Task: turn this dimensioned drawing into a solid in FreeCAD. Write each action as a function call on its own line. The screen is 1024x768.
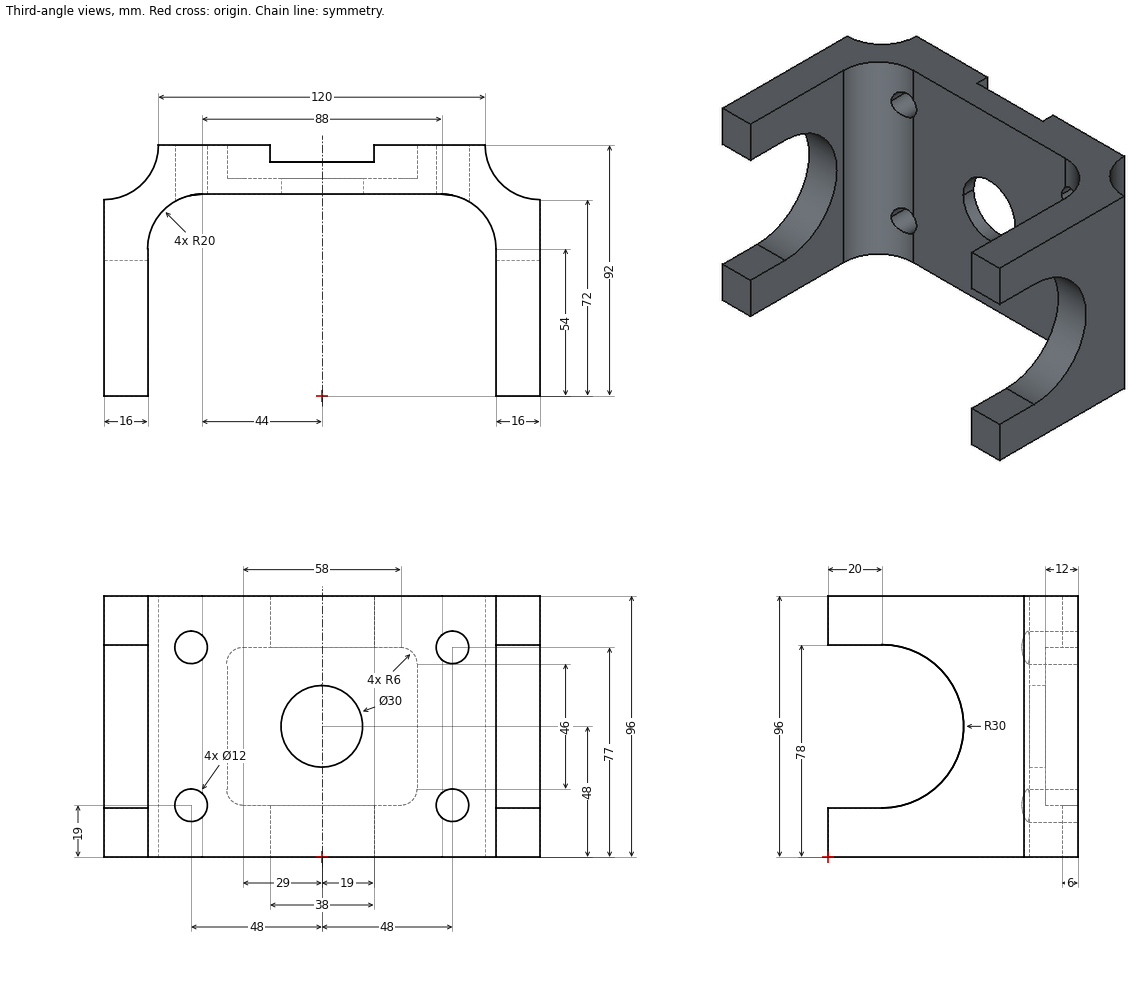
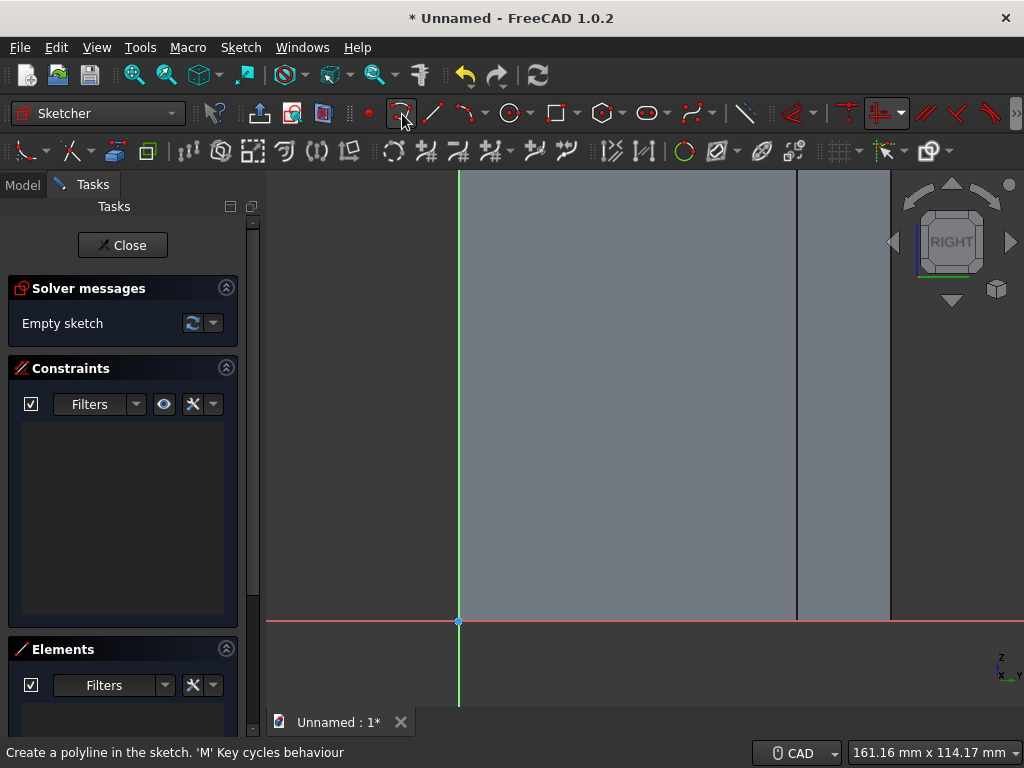
click(553, 255)
click(459, 255)
click(468, 537)
click(553, 537)
right_click(553, 537)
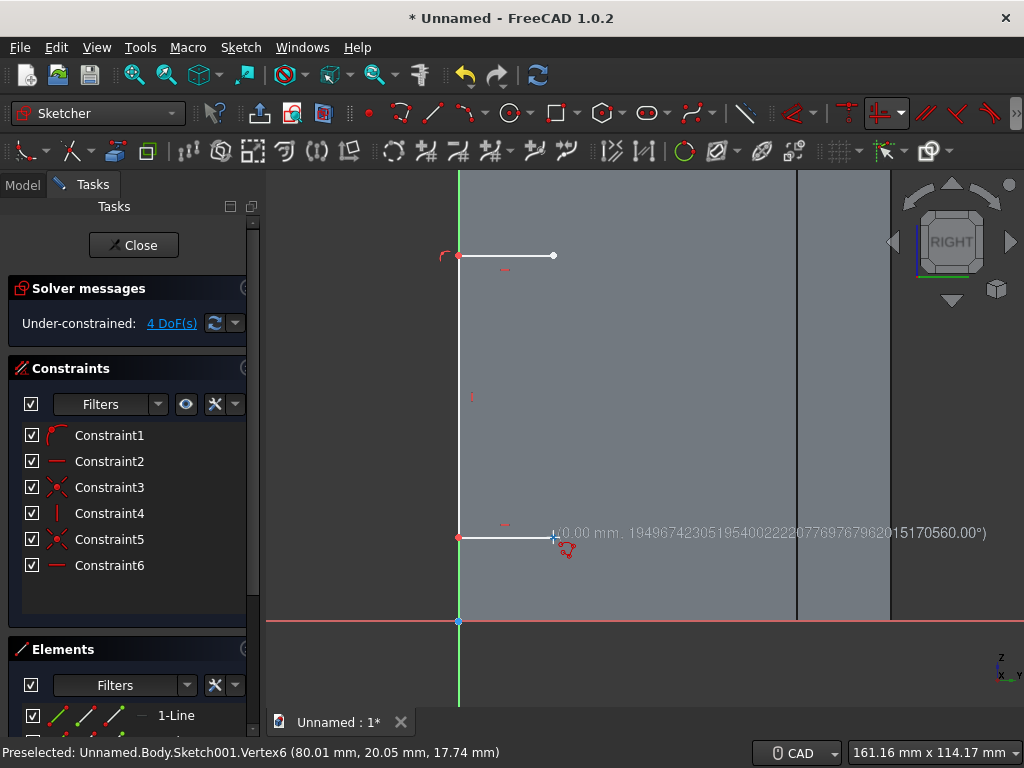
click(466, 114)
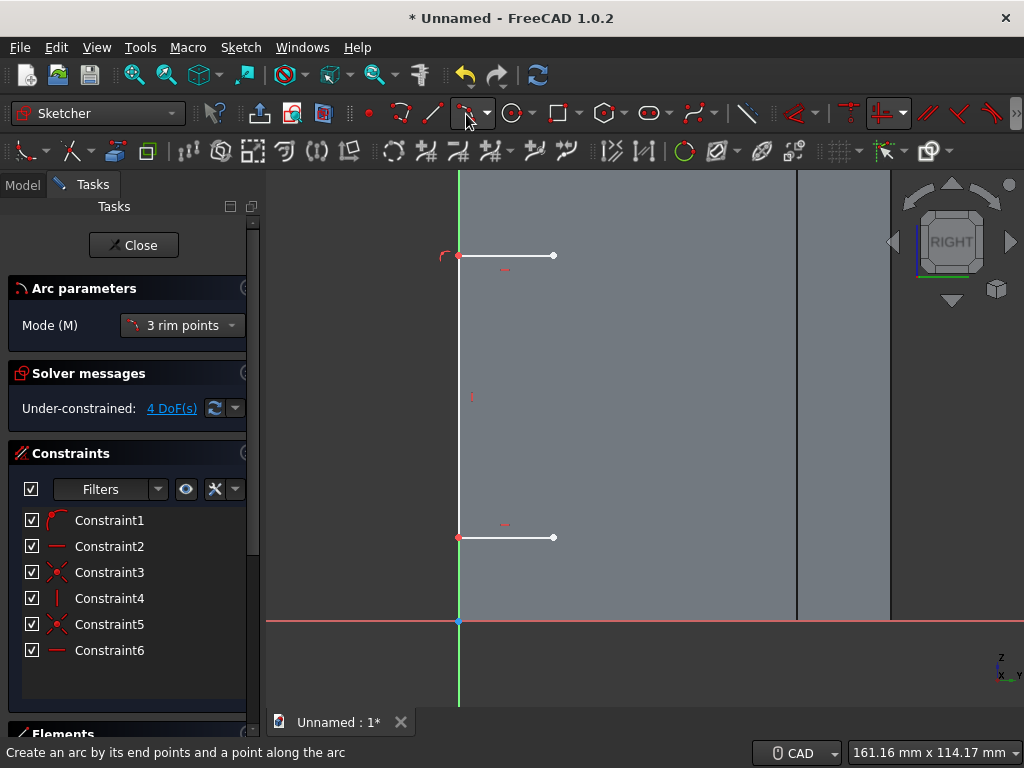
click(553, 538)
click(553, 256)
click(694, 396)
key(Escape)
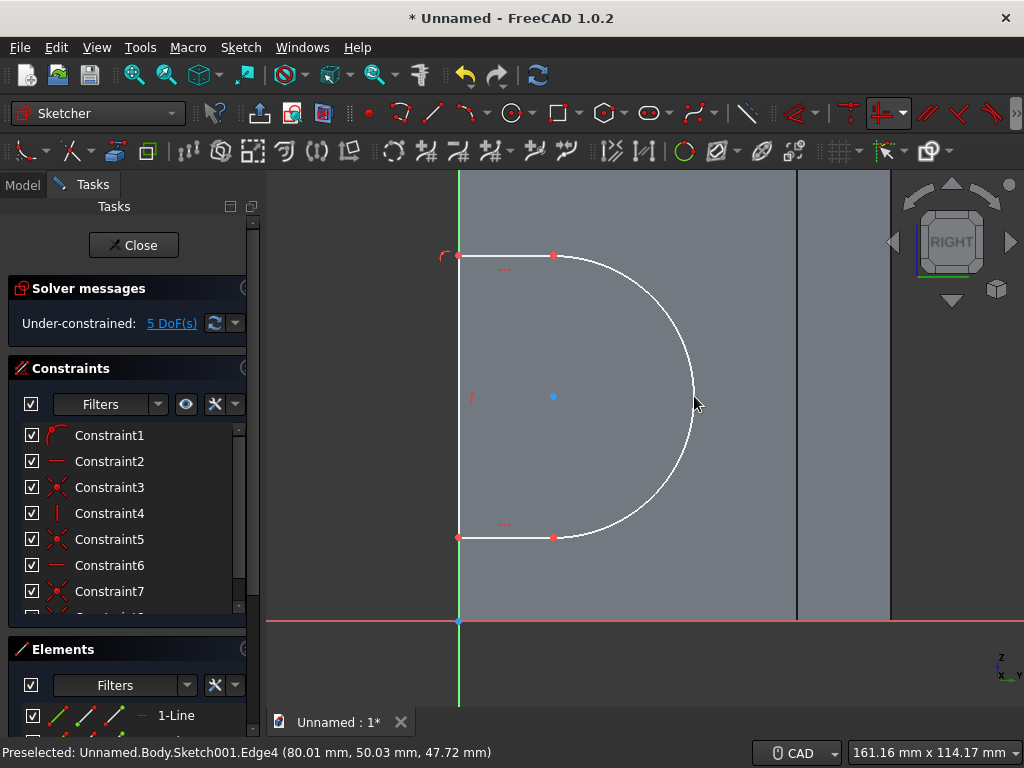
click(525, 256)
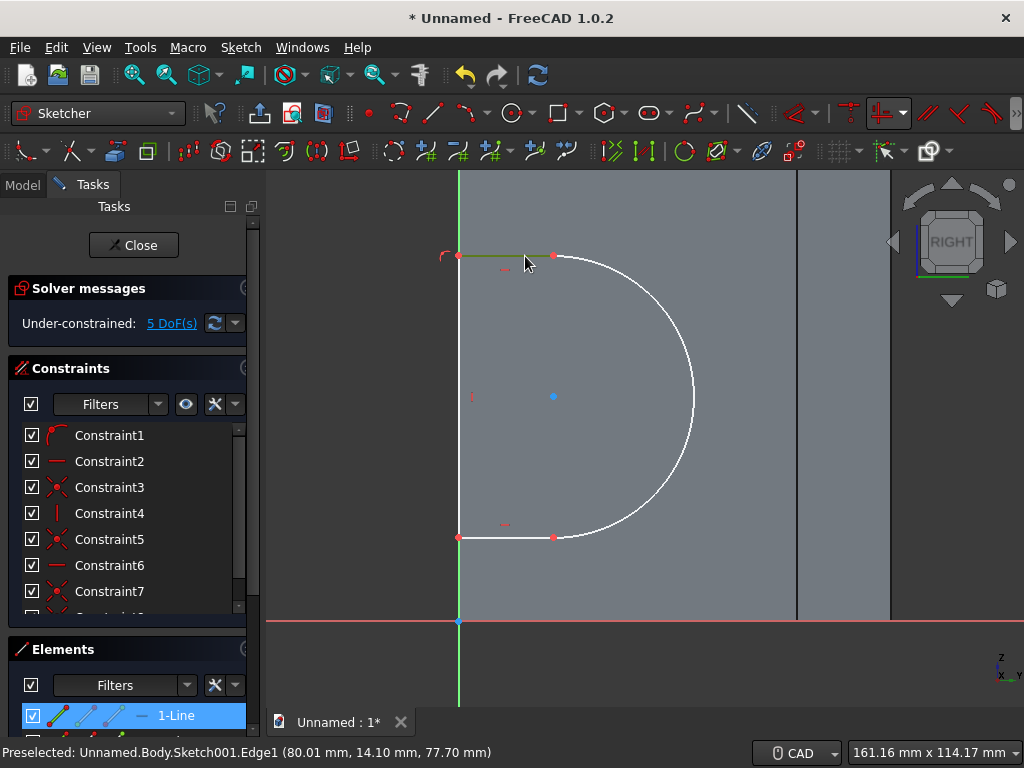
click(667, 480)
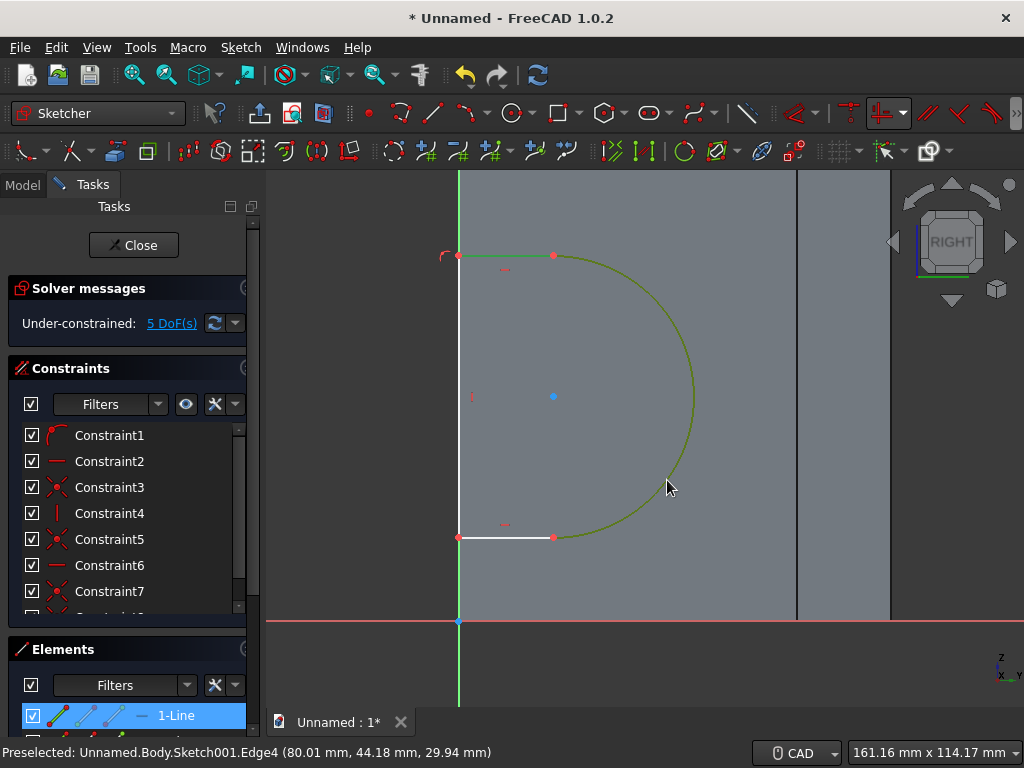
click(992, 114)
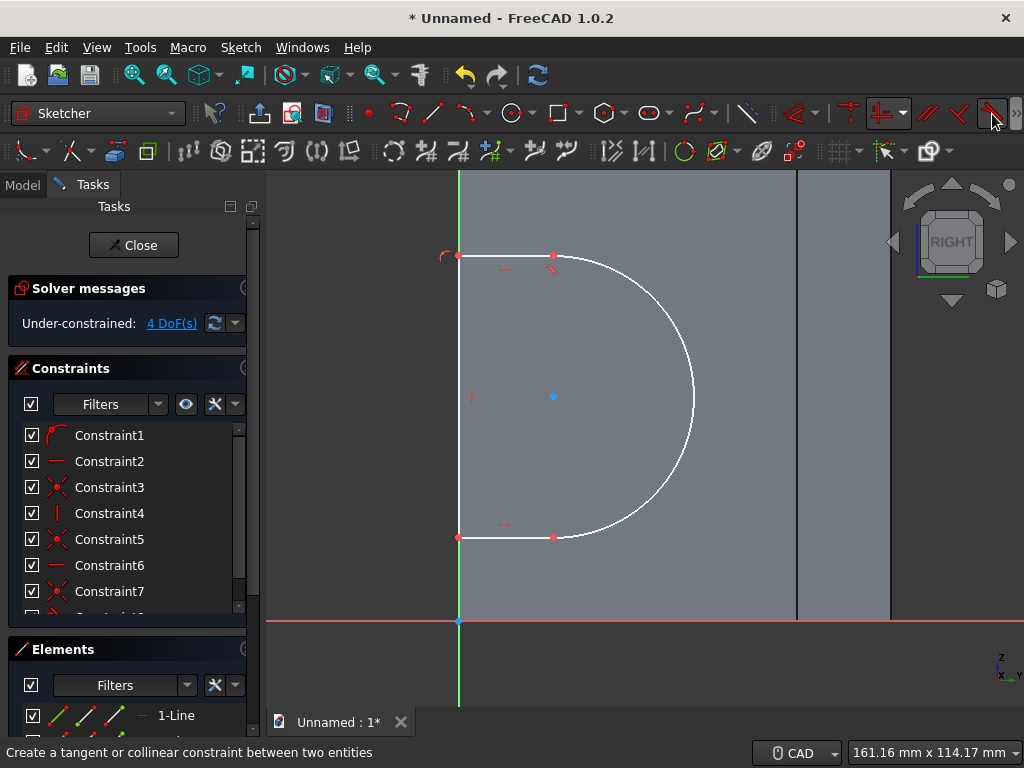
click(487, 538)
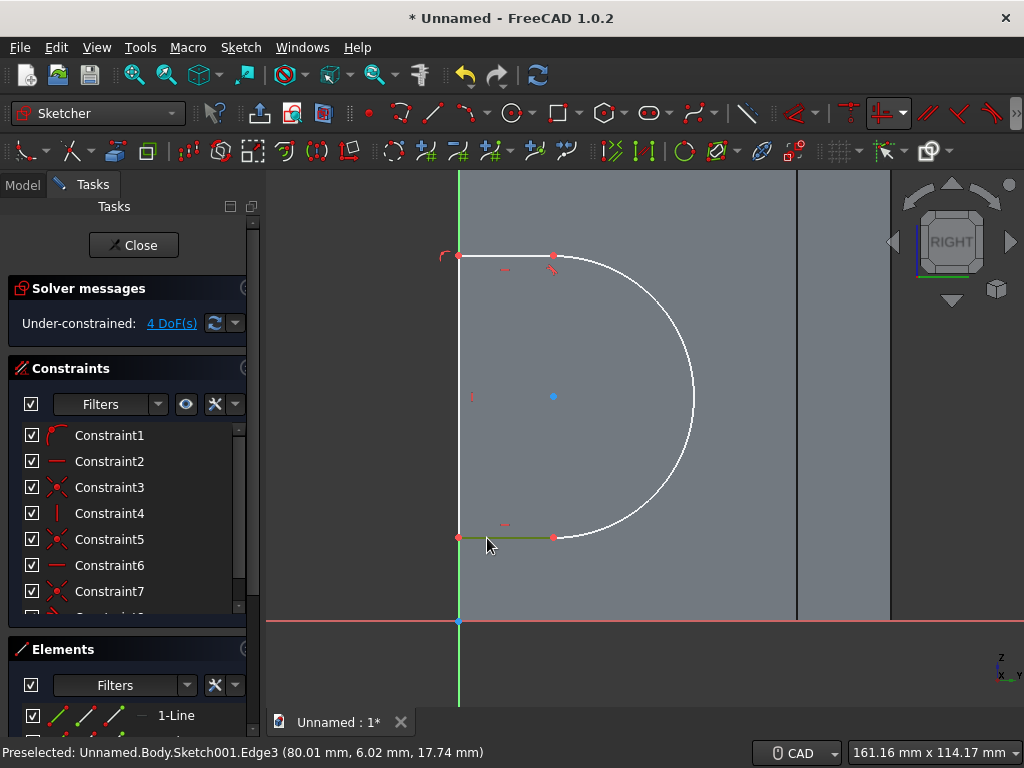
click(667, 480)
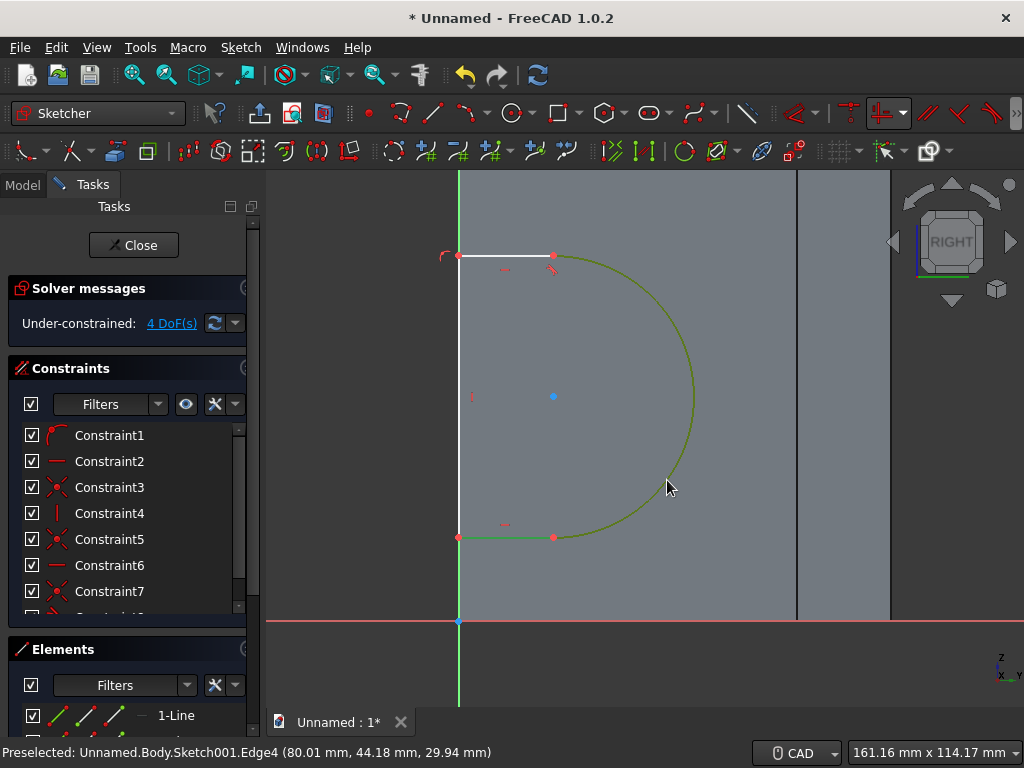
click(992, 114)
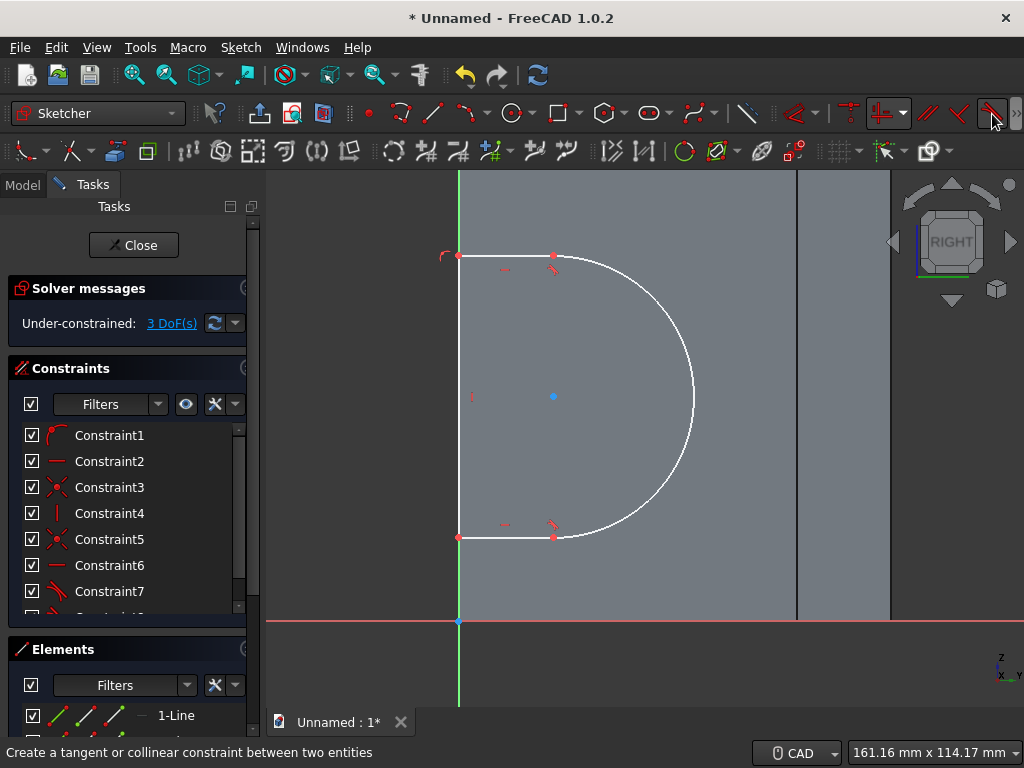
click(794, 114)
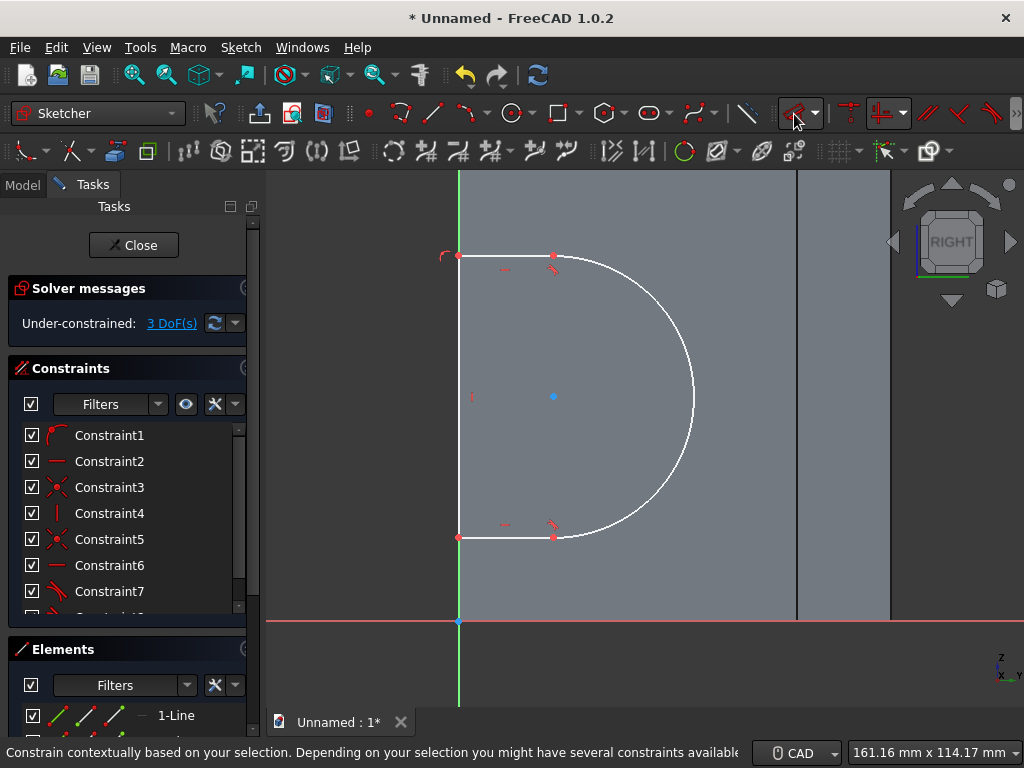
click(667, 480)
click(693, 499)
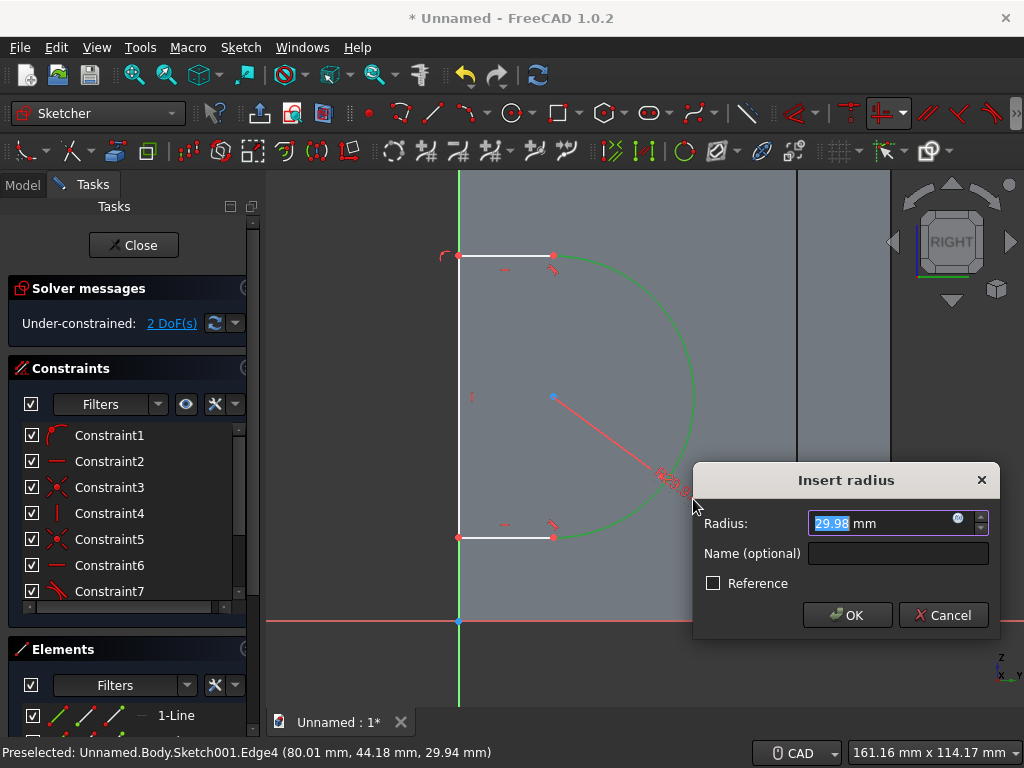
text(30)
key(Return)